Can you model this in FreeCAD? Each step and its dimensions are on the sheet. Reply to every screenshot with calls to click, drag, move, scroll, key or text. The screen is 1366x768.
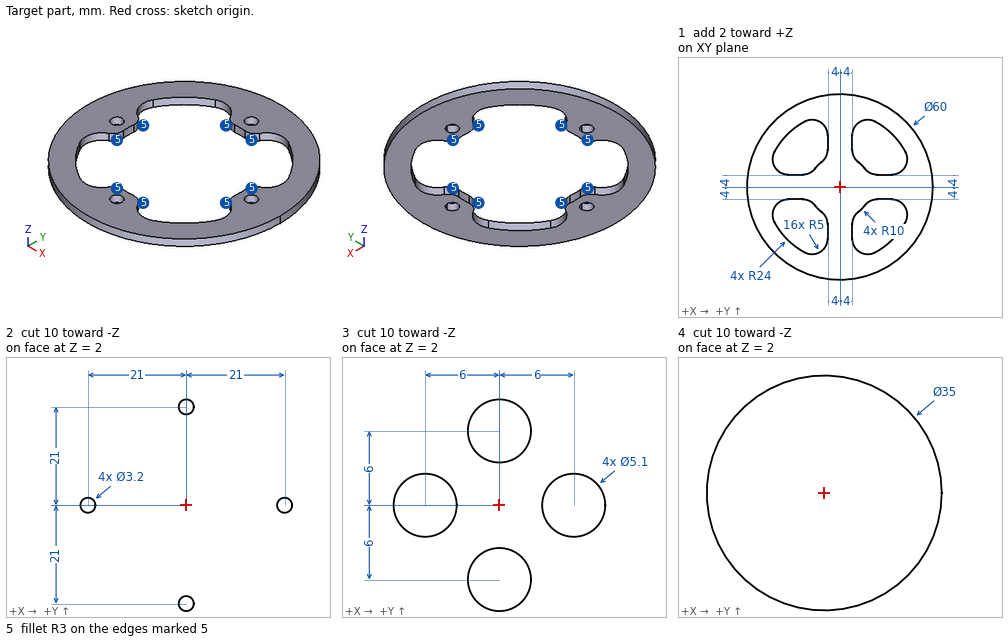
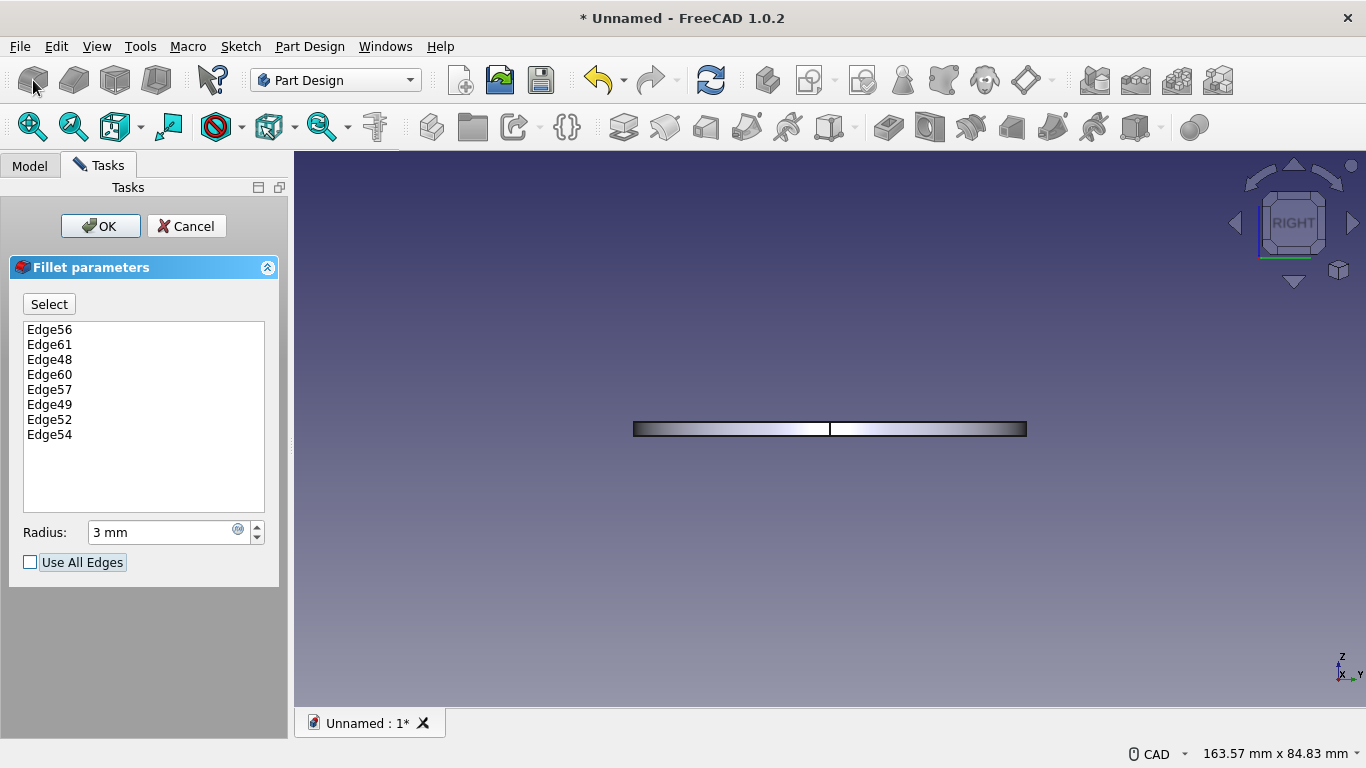
click(101, 226)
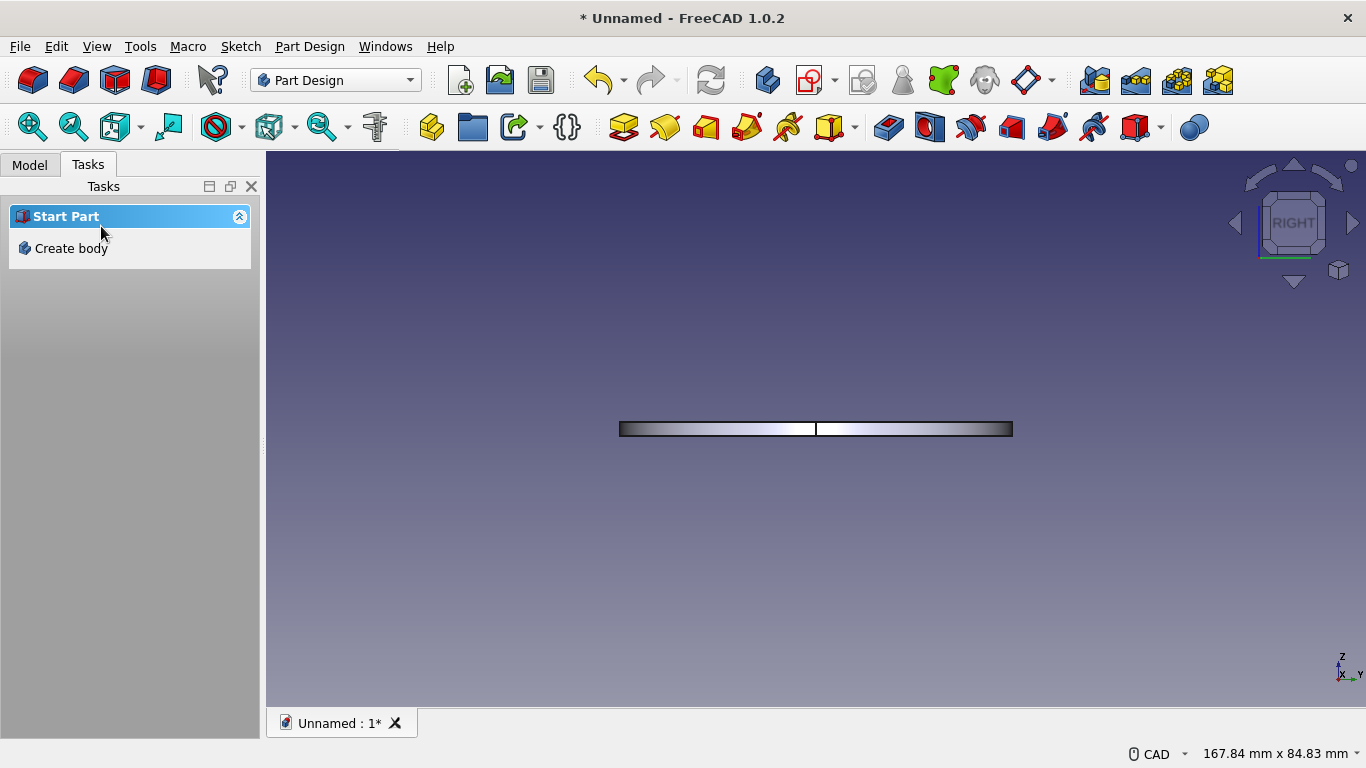
key(0)